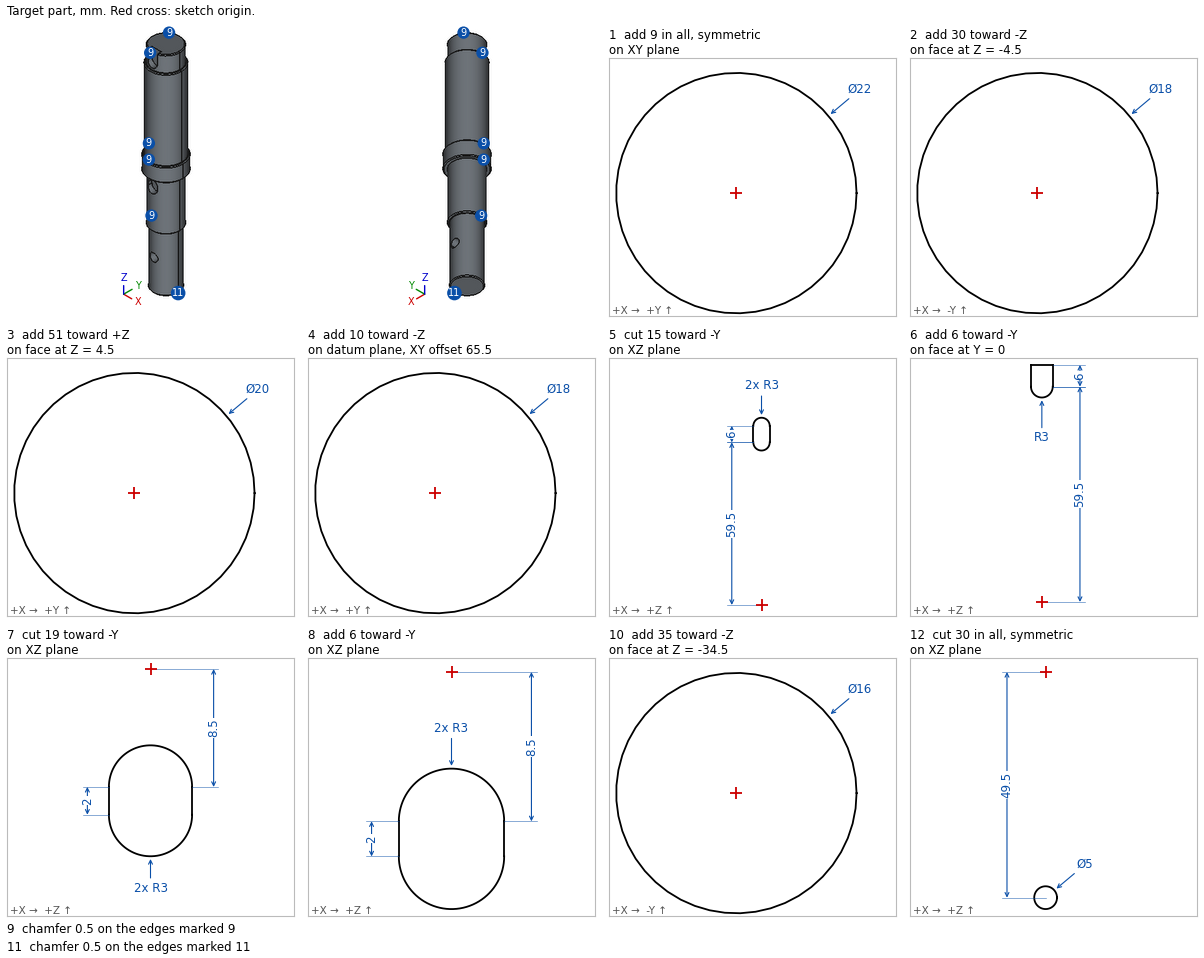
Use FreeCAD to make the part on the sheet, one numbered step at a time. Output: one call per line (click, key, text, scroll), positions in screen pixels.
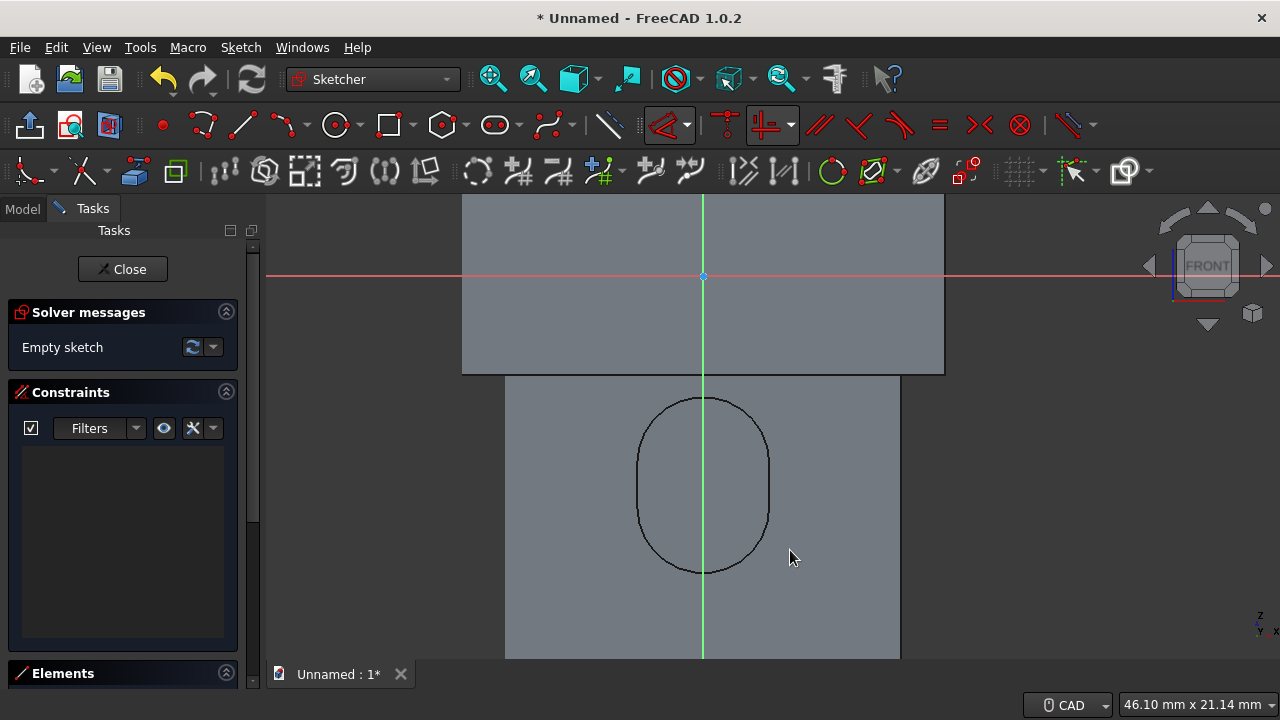
click(496, 126)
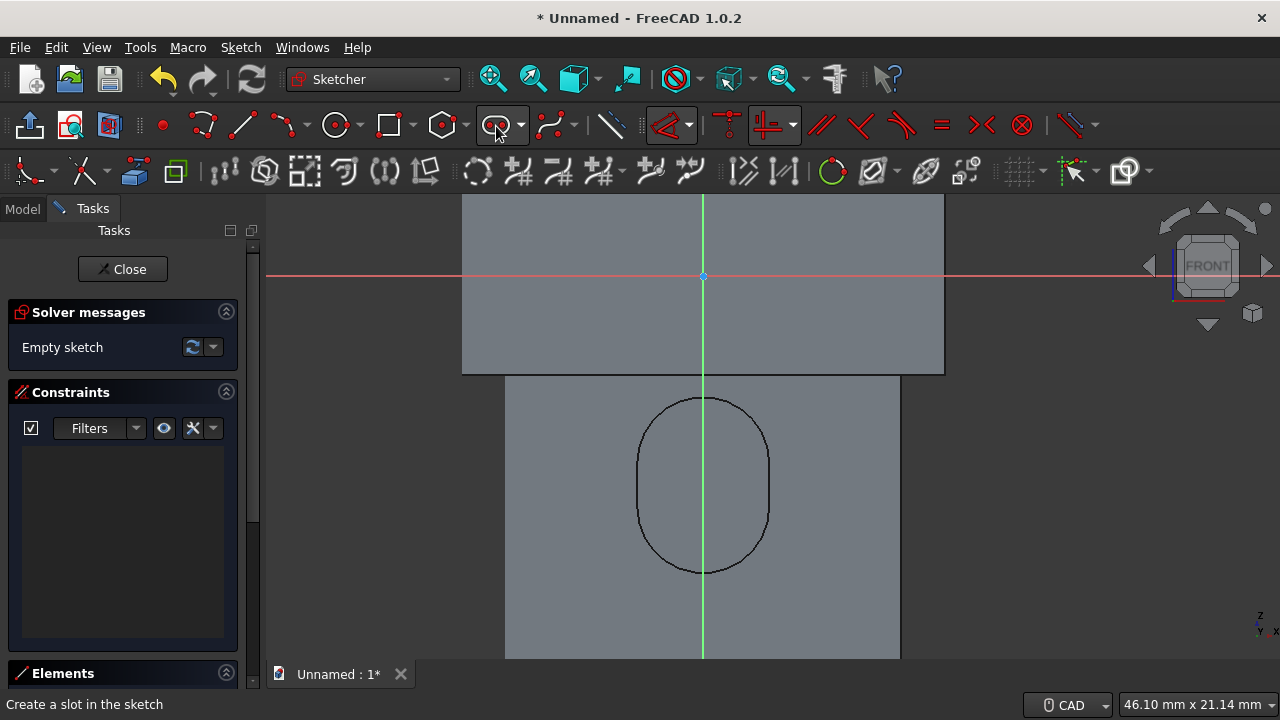
click(703, 507)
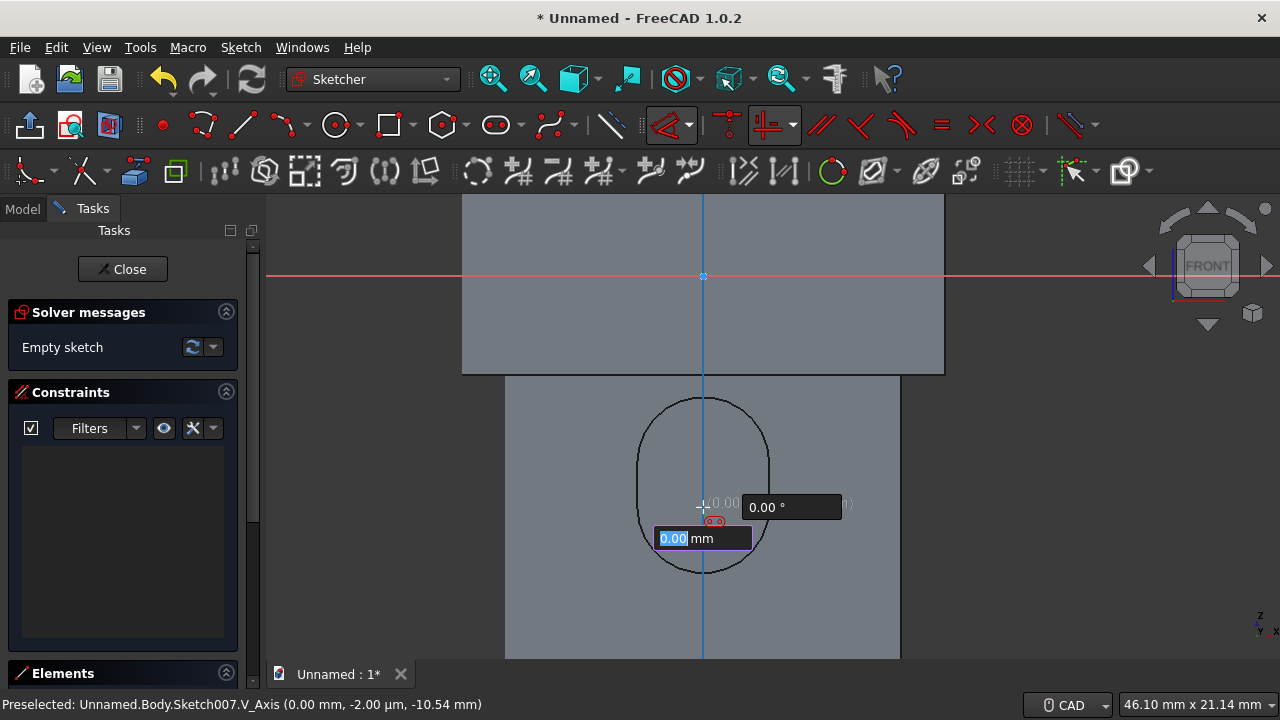
click(712, 463)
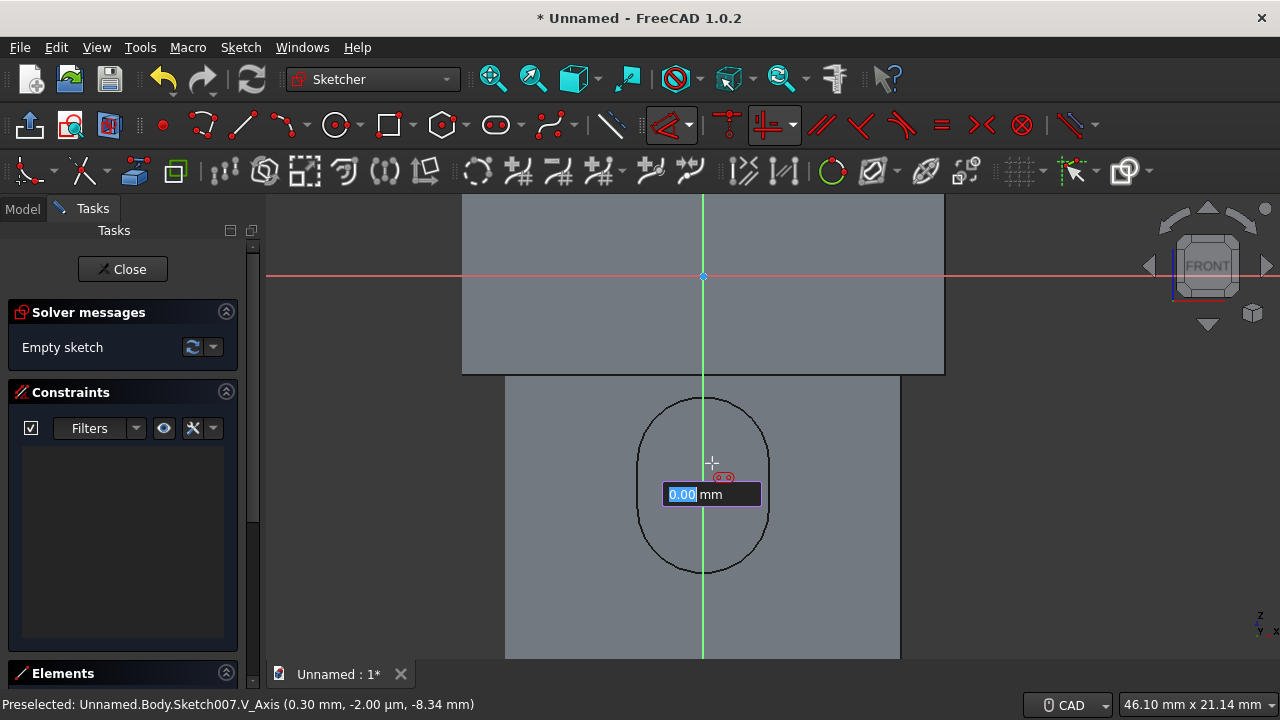
click(769, 485)
key(Escape)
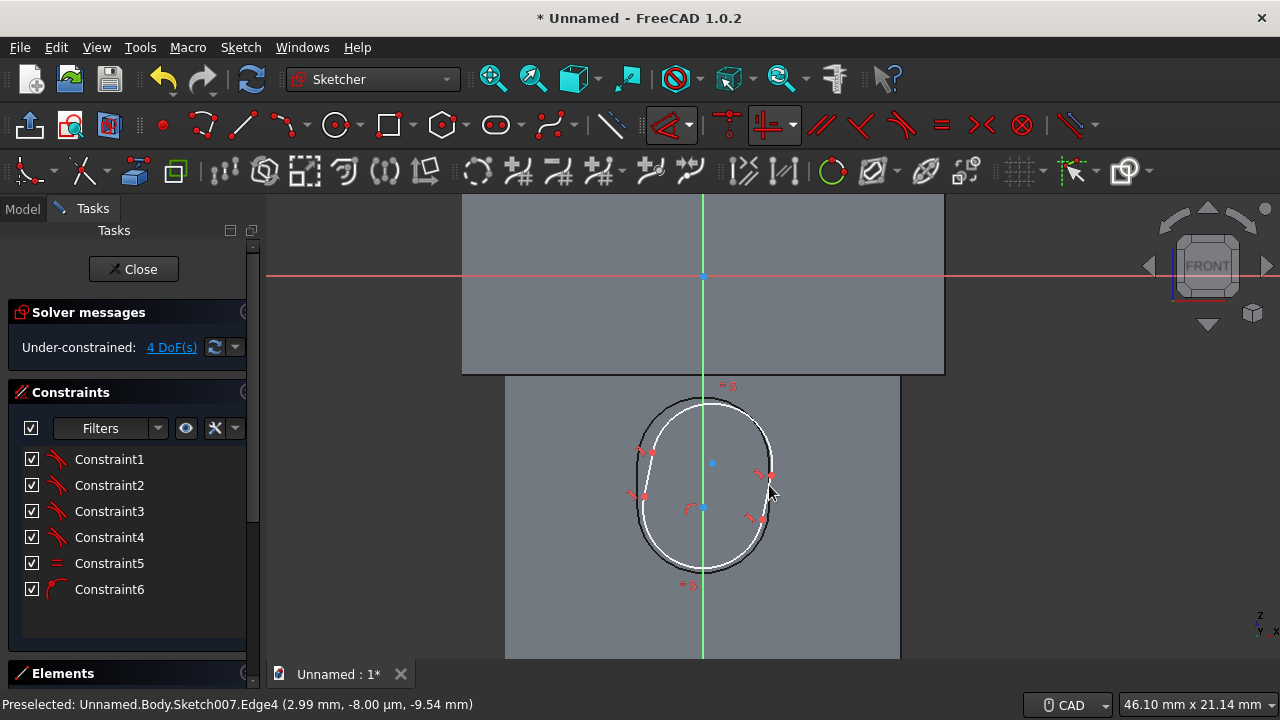
click(647, 483)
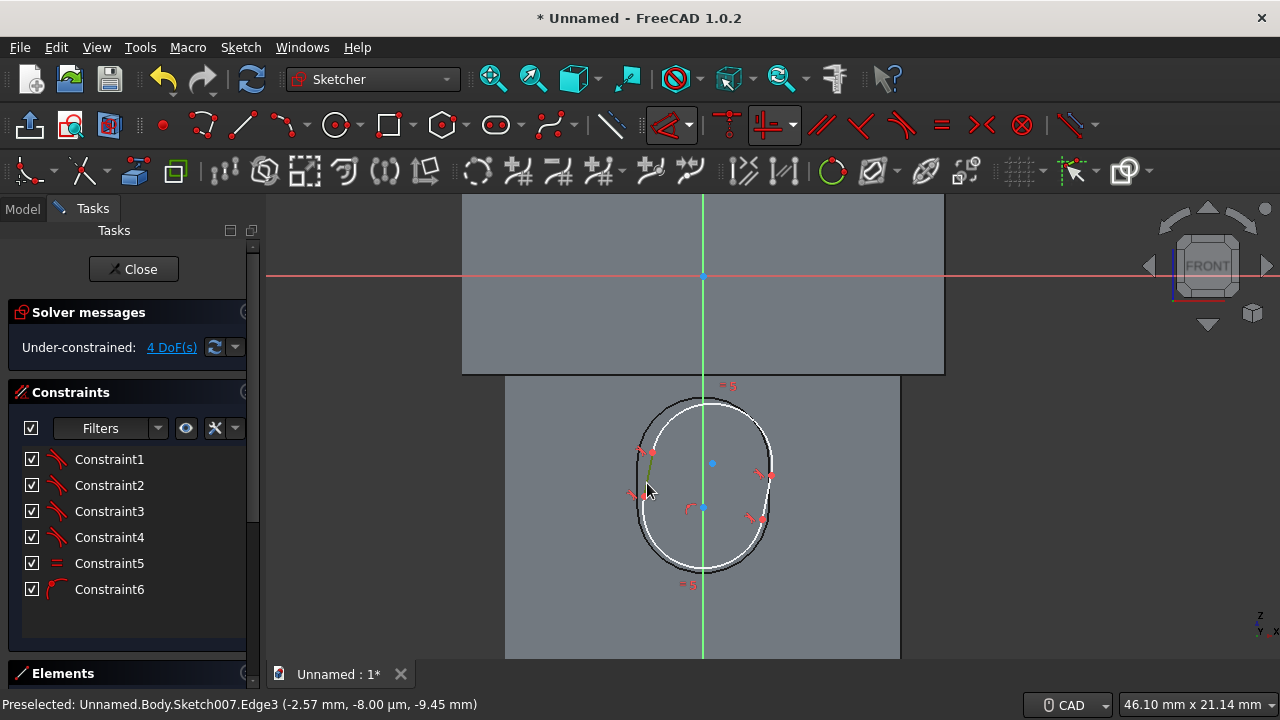
key(v)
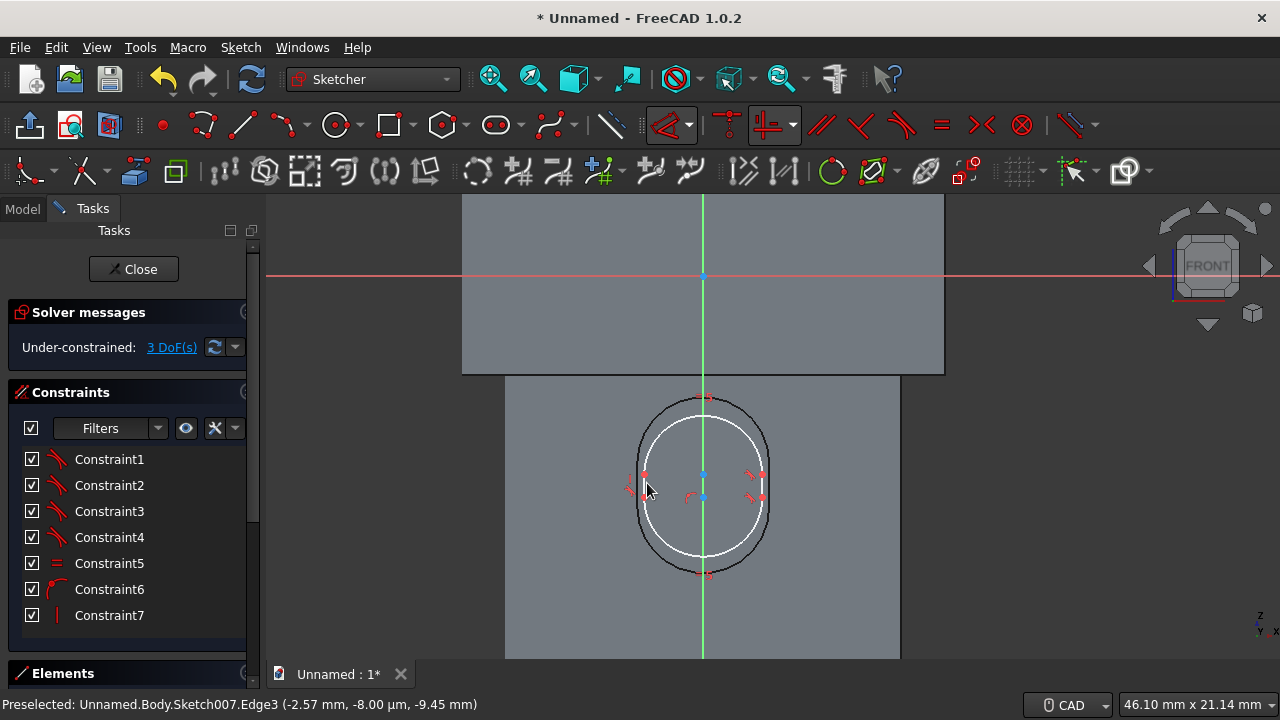
click(669, 545)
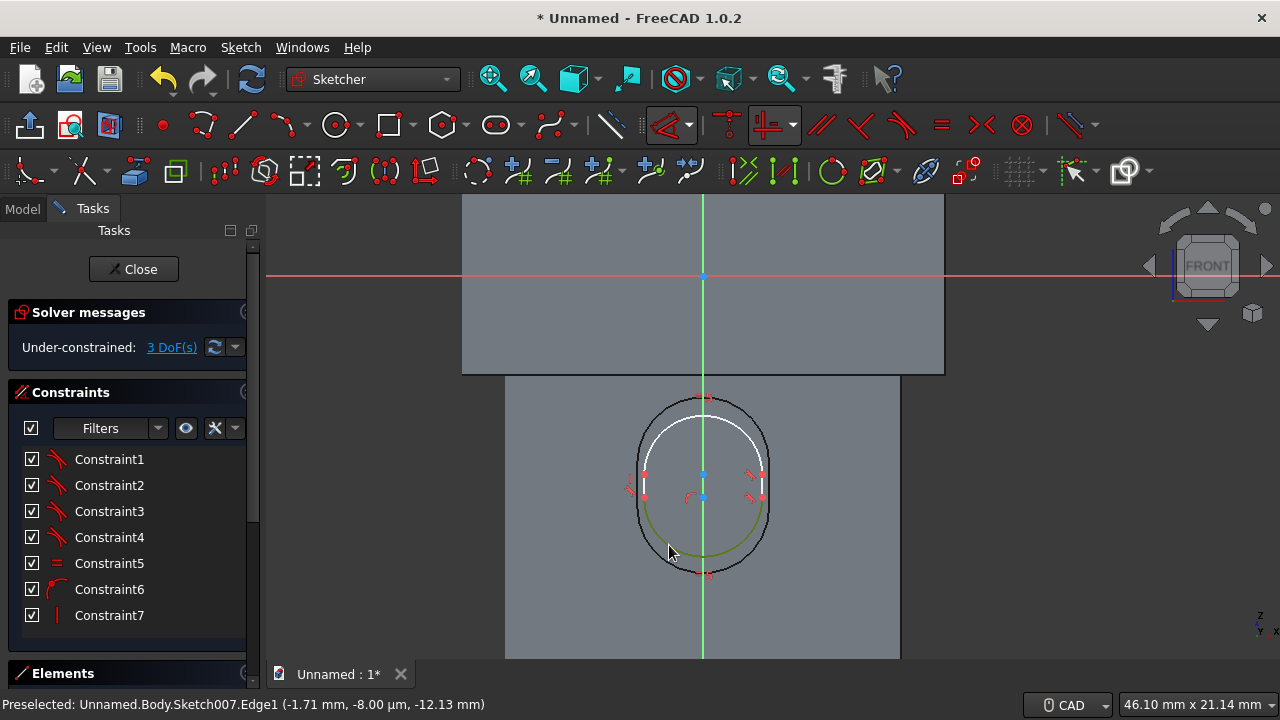
click(692, 126)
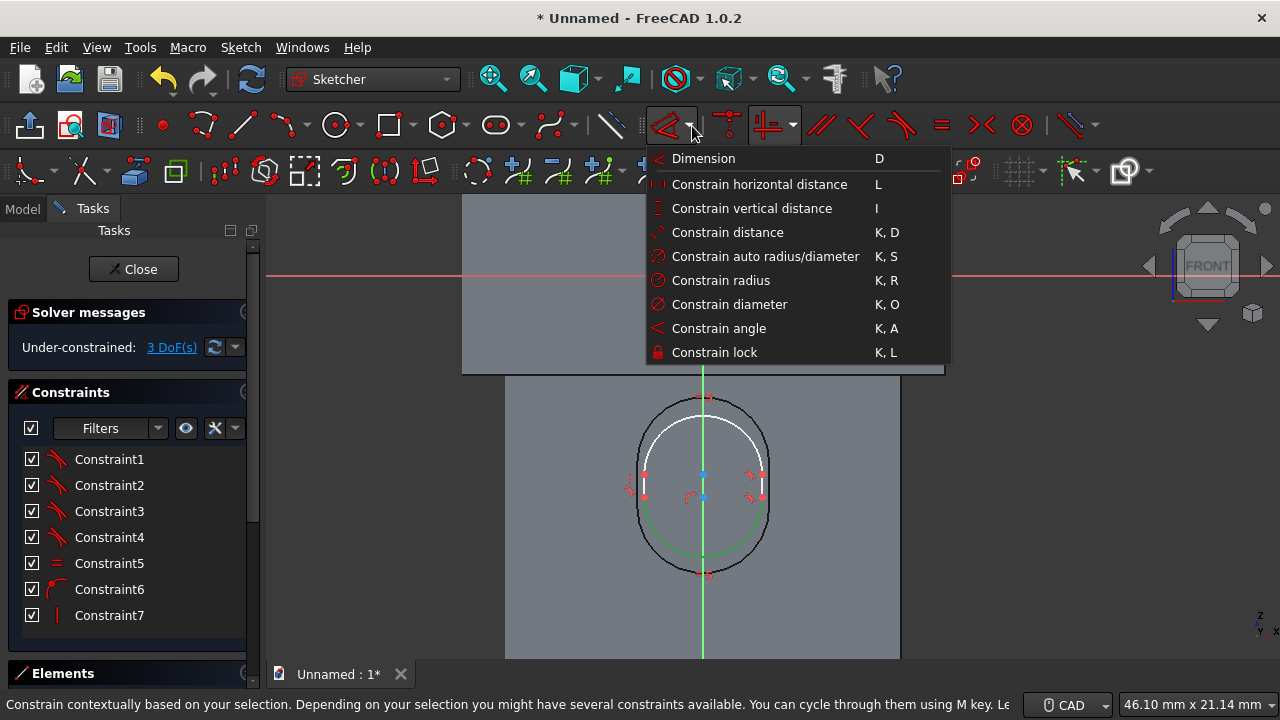
click(799, 280)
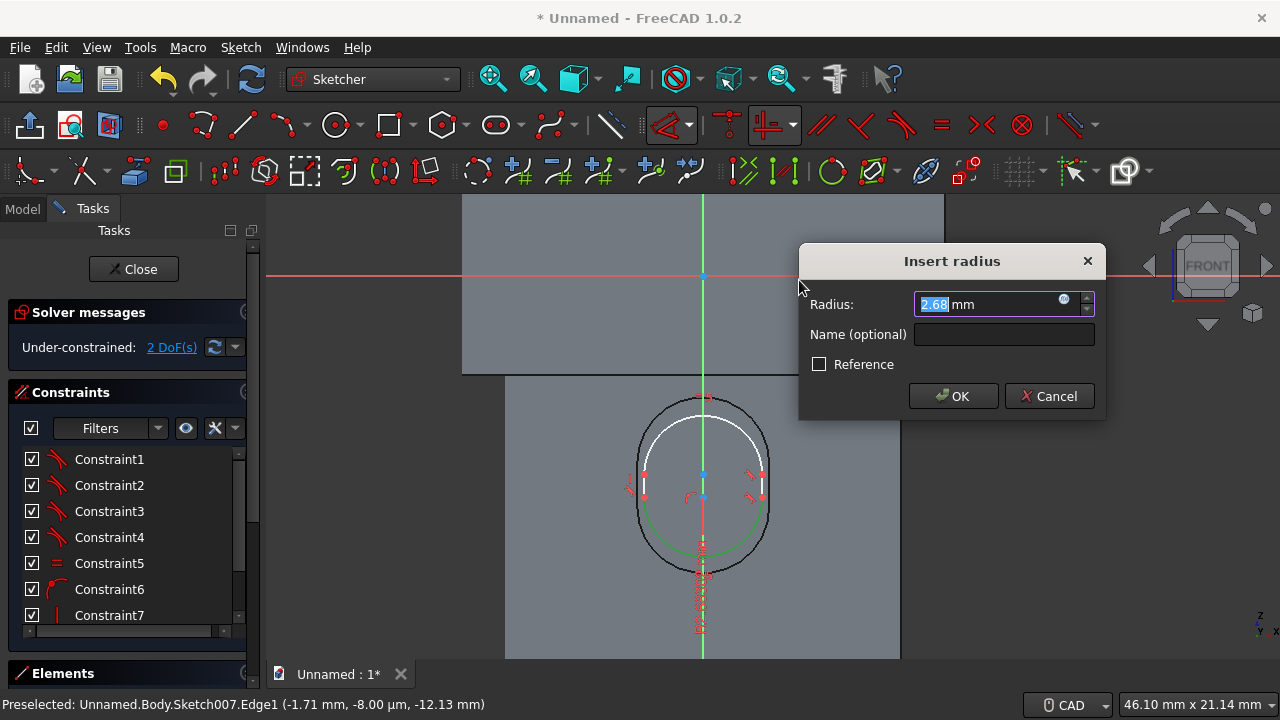
text(3)
key(Return)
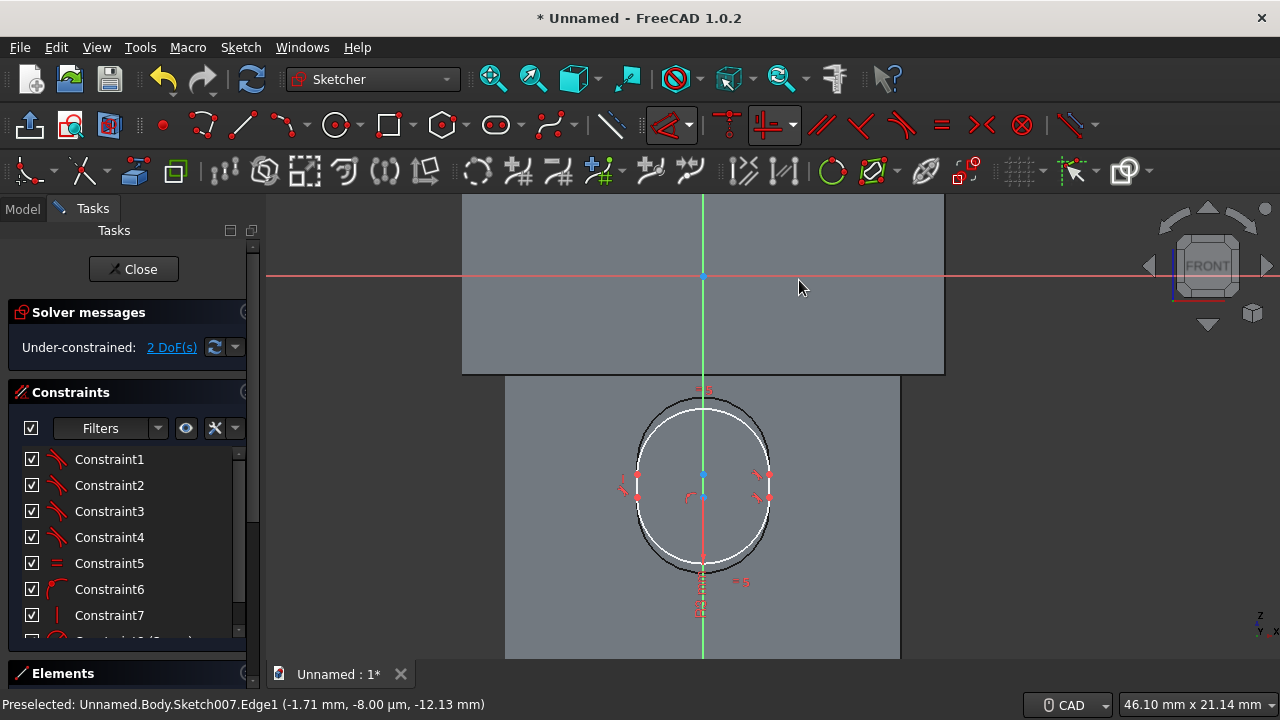
scroll(637, 489, up, 3)